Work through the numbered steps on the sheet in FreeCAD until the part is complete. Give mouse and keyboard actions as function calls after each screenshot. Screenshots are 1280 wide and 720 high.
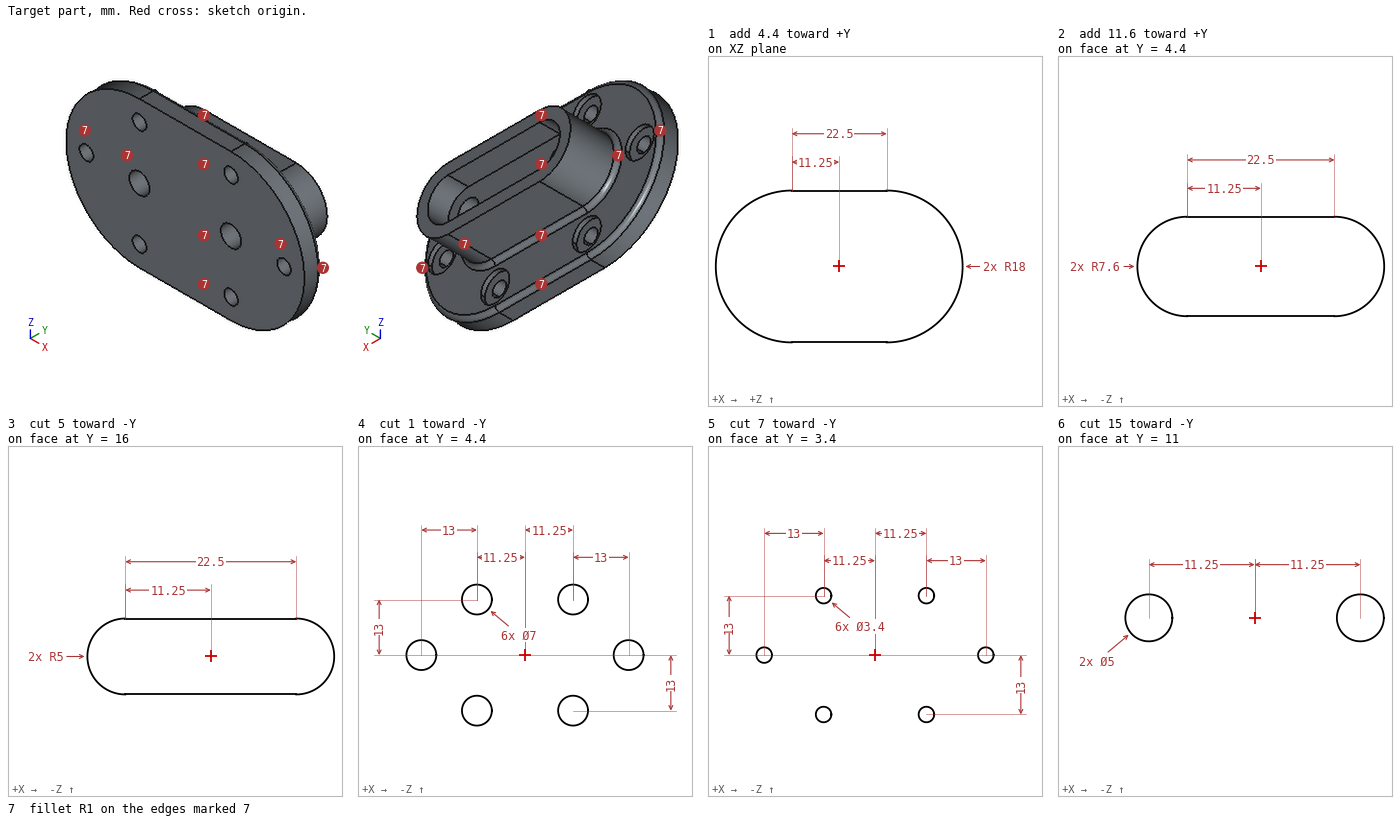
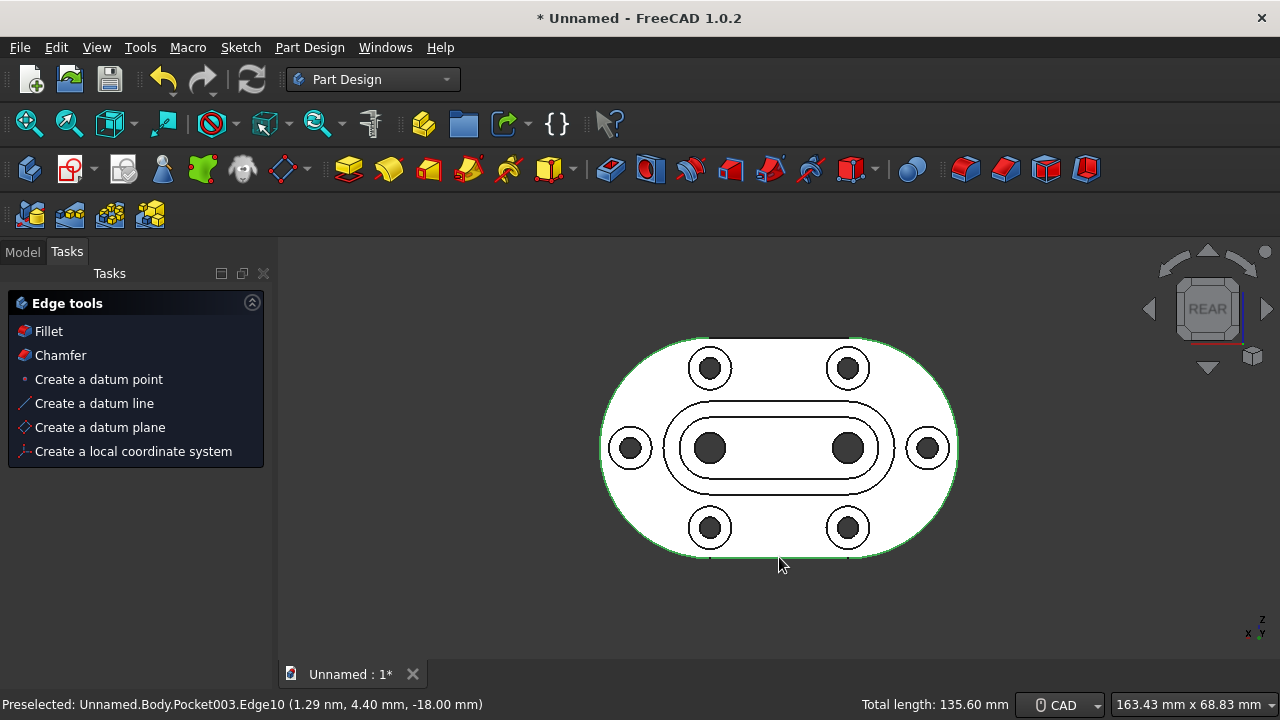
key(0)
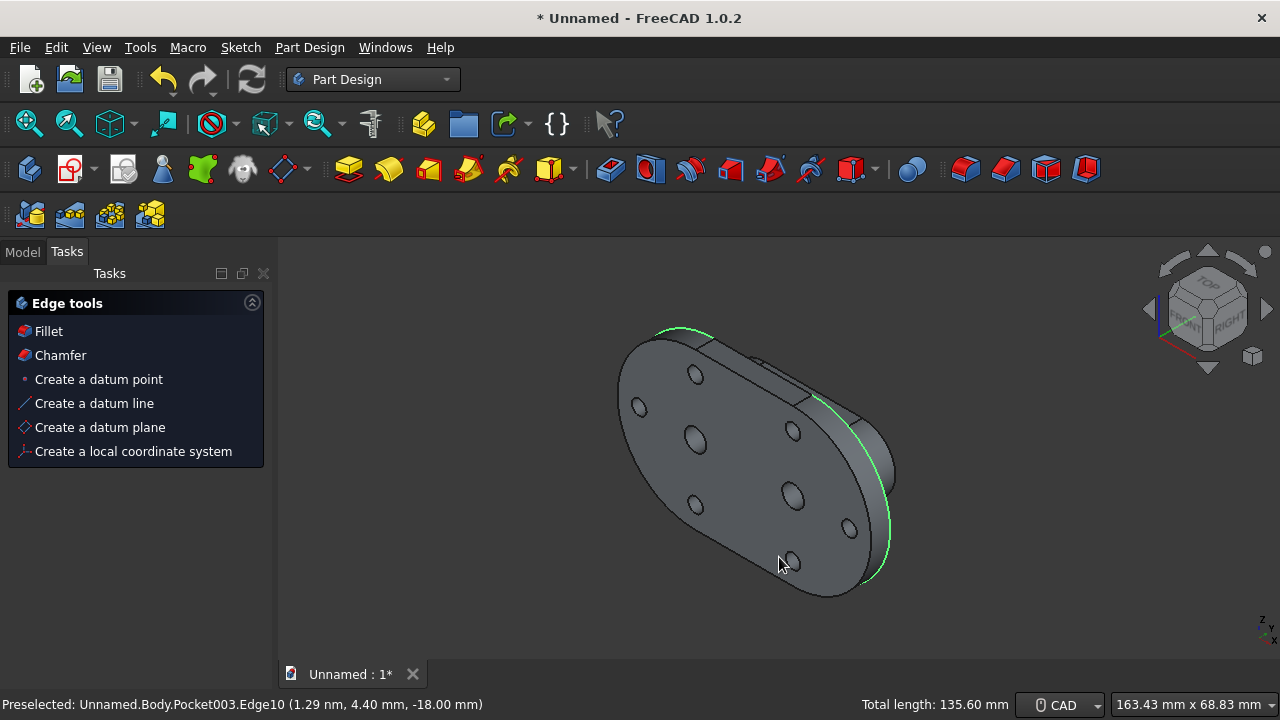
key(2)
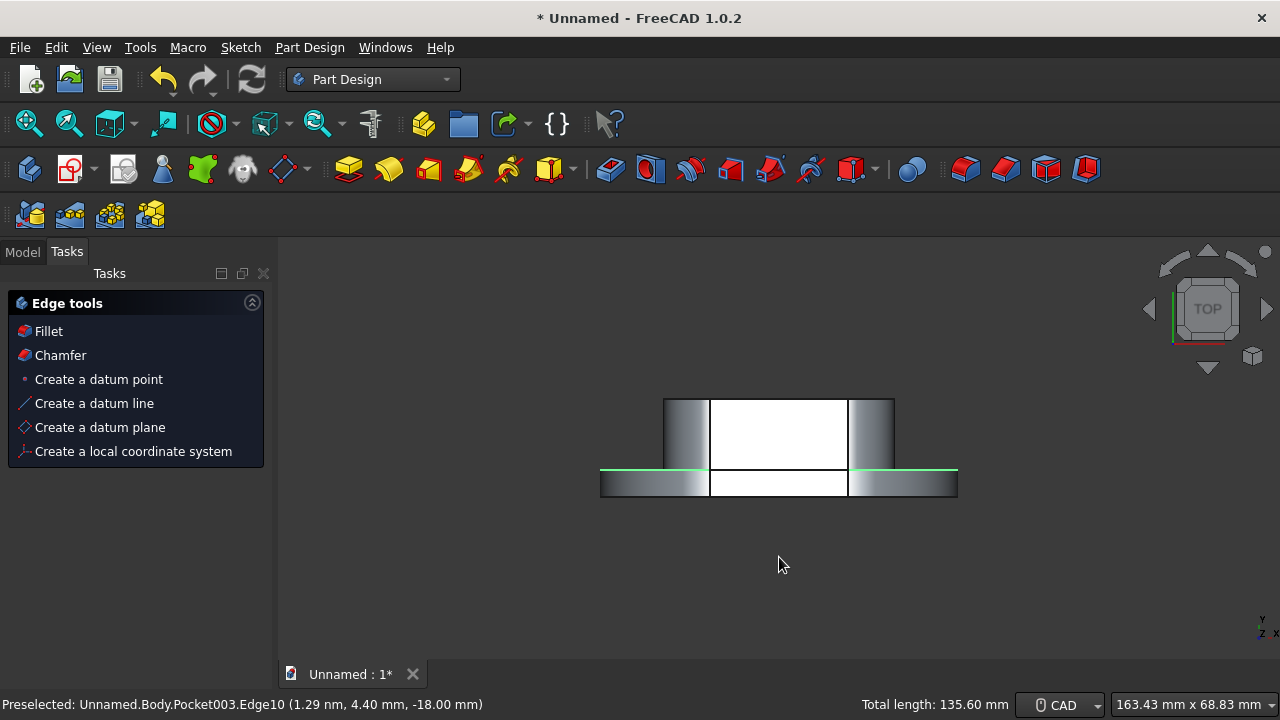
click(30, 124)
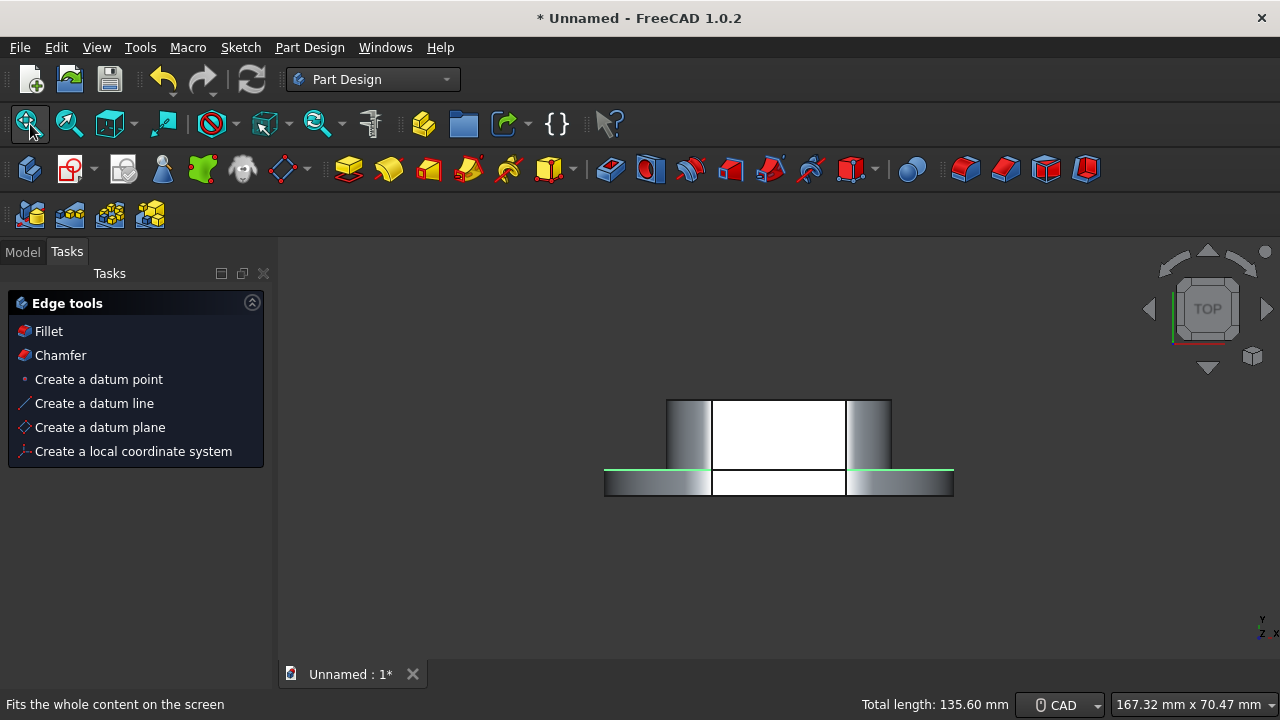
click(779, 469, ctrl)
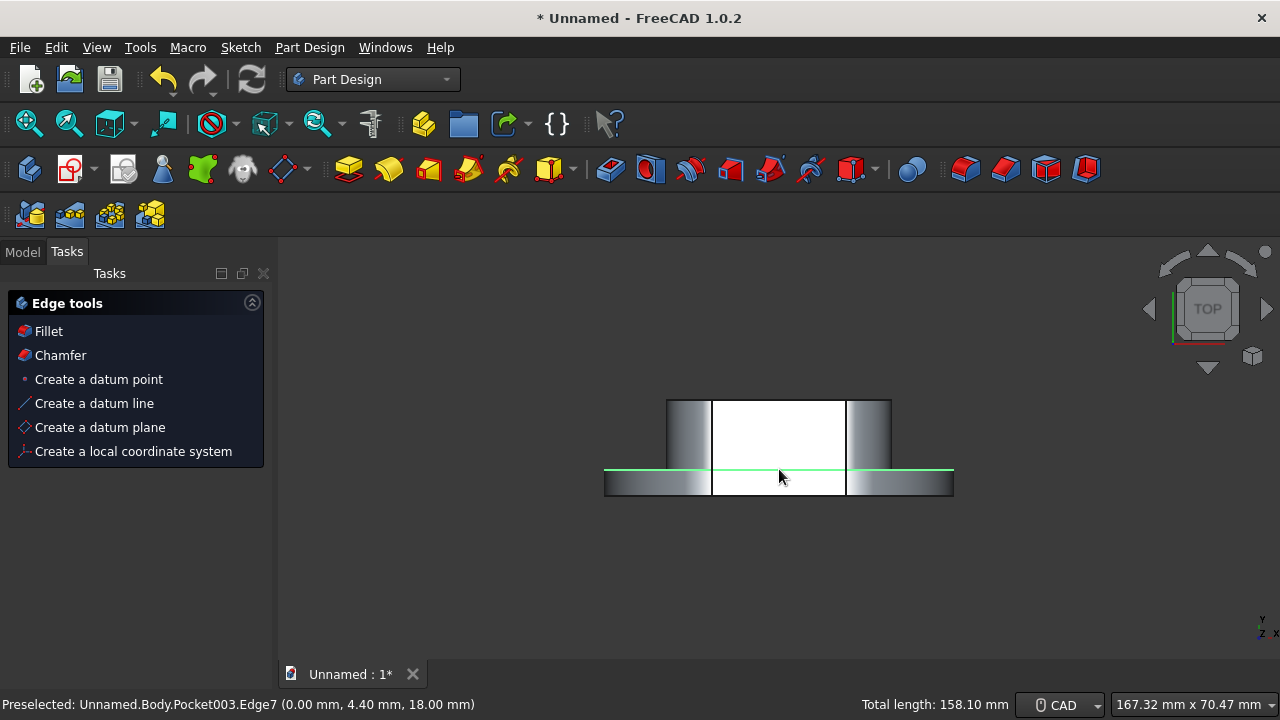
key(1)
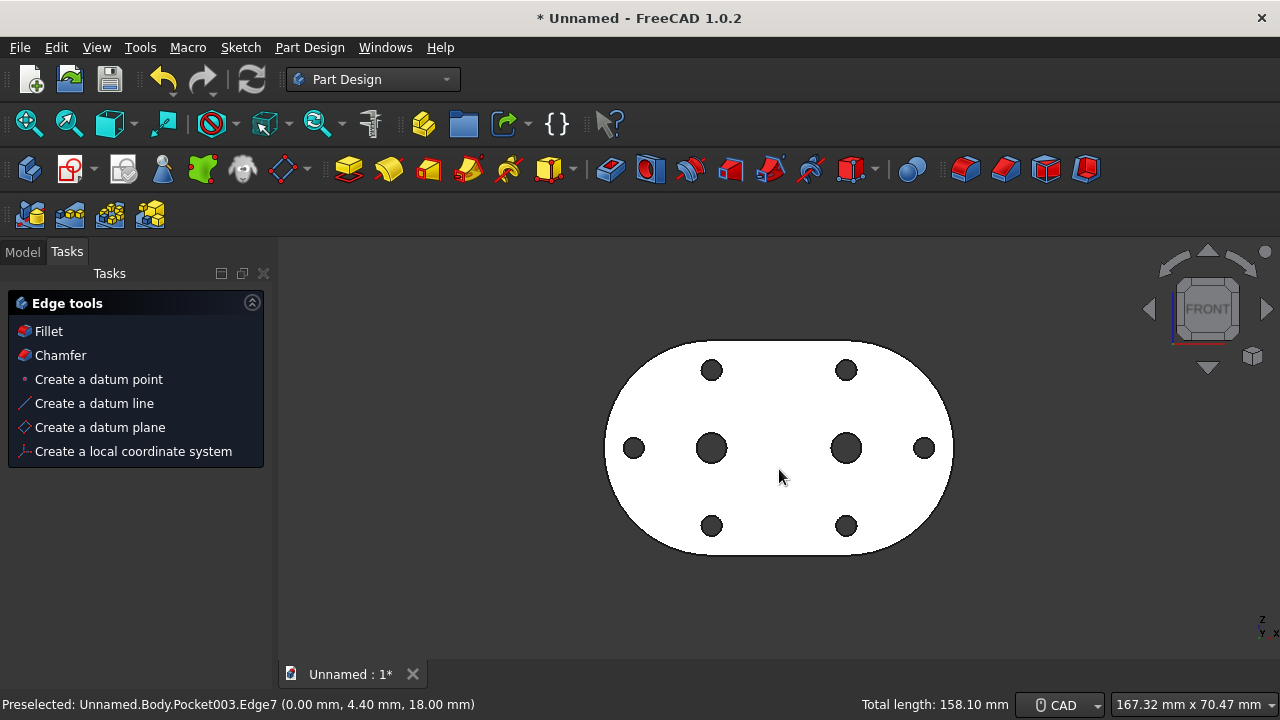
key(3)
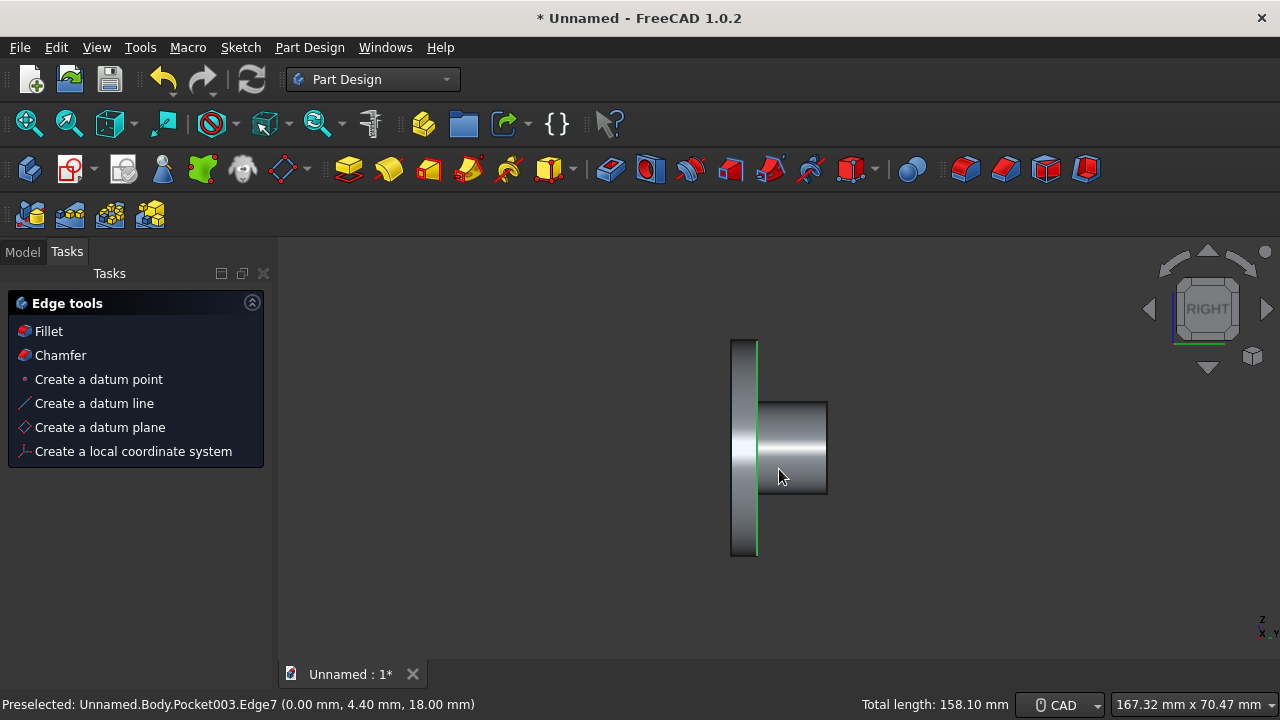
key(5)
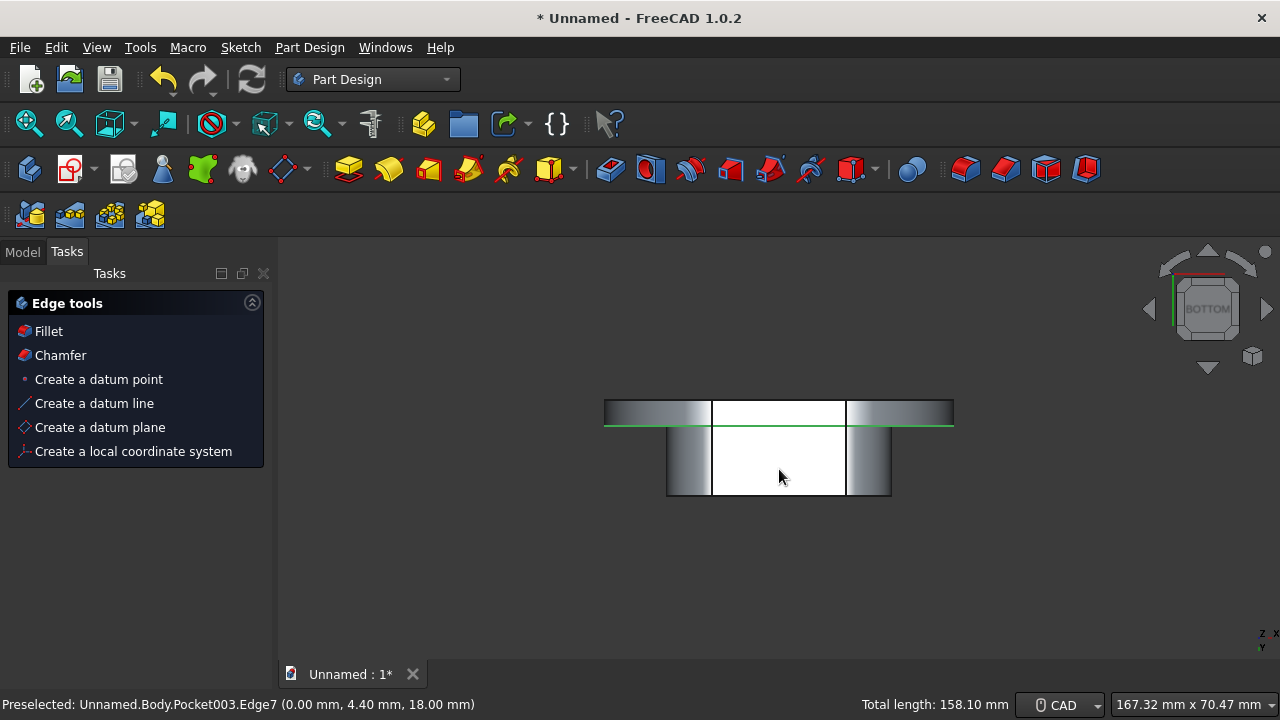
click(30, 124)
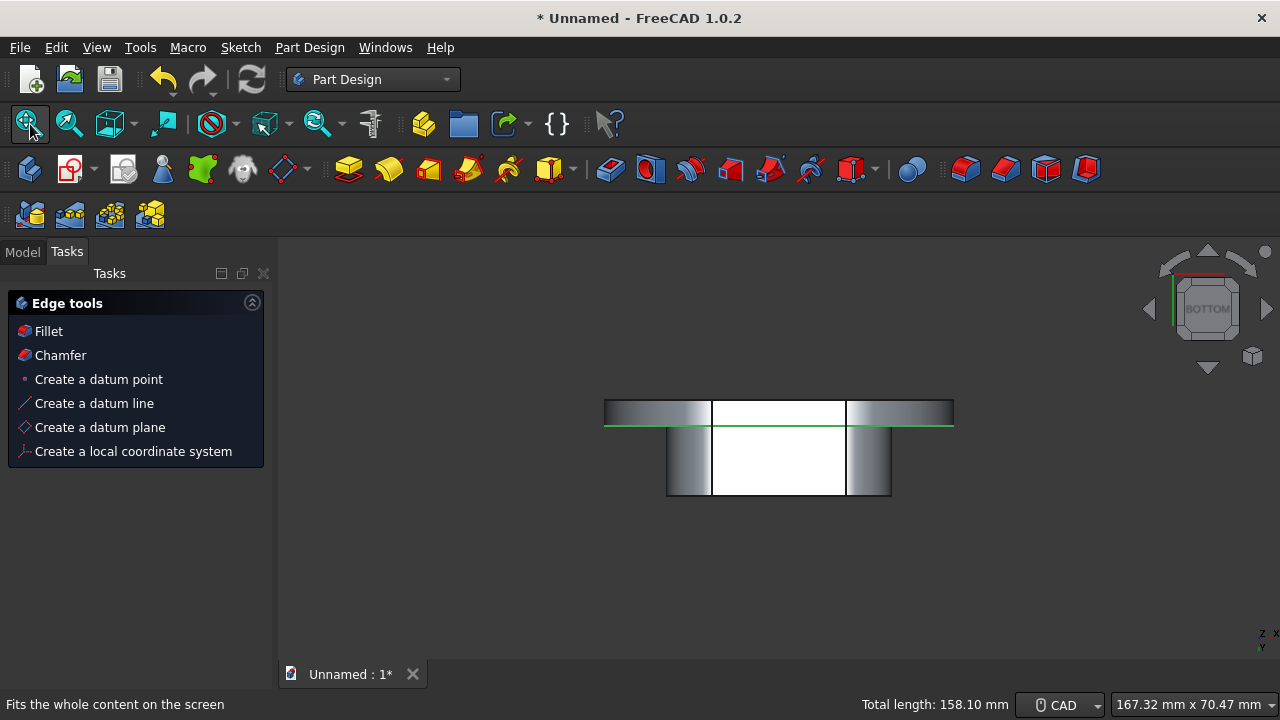
key(4)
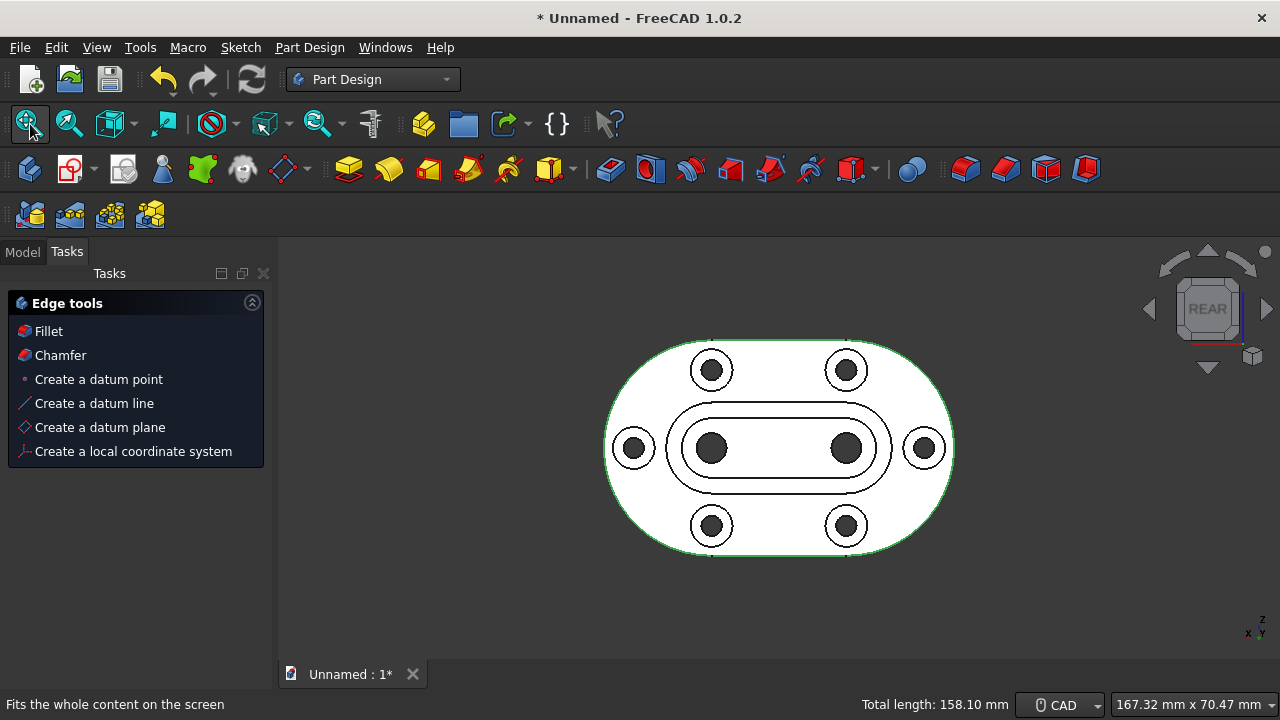
key(6)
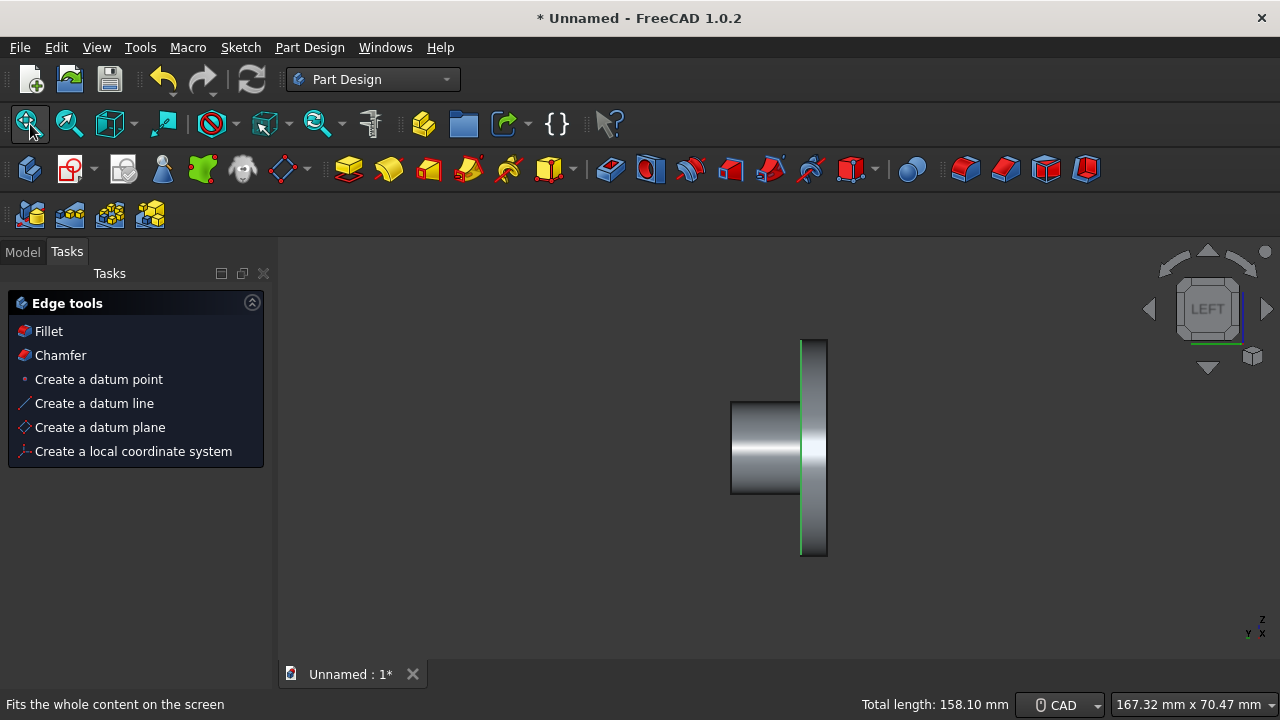
key(v)
key(3)